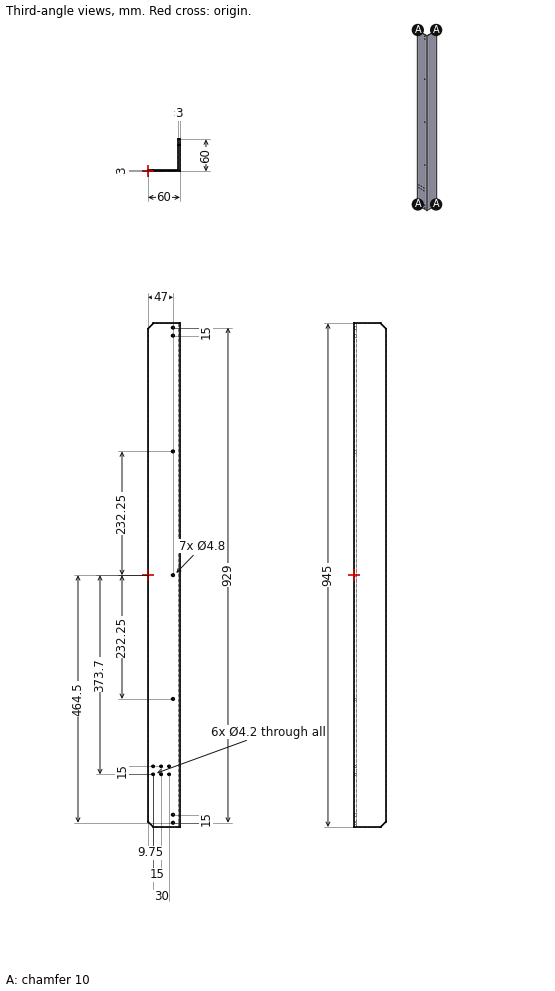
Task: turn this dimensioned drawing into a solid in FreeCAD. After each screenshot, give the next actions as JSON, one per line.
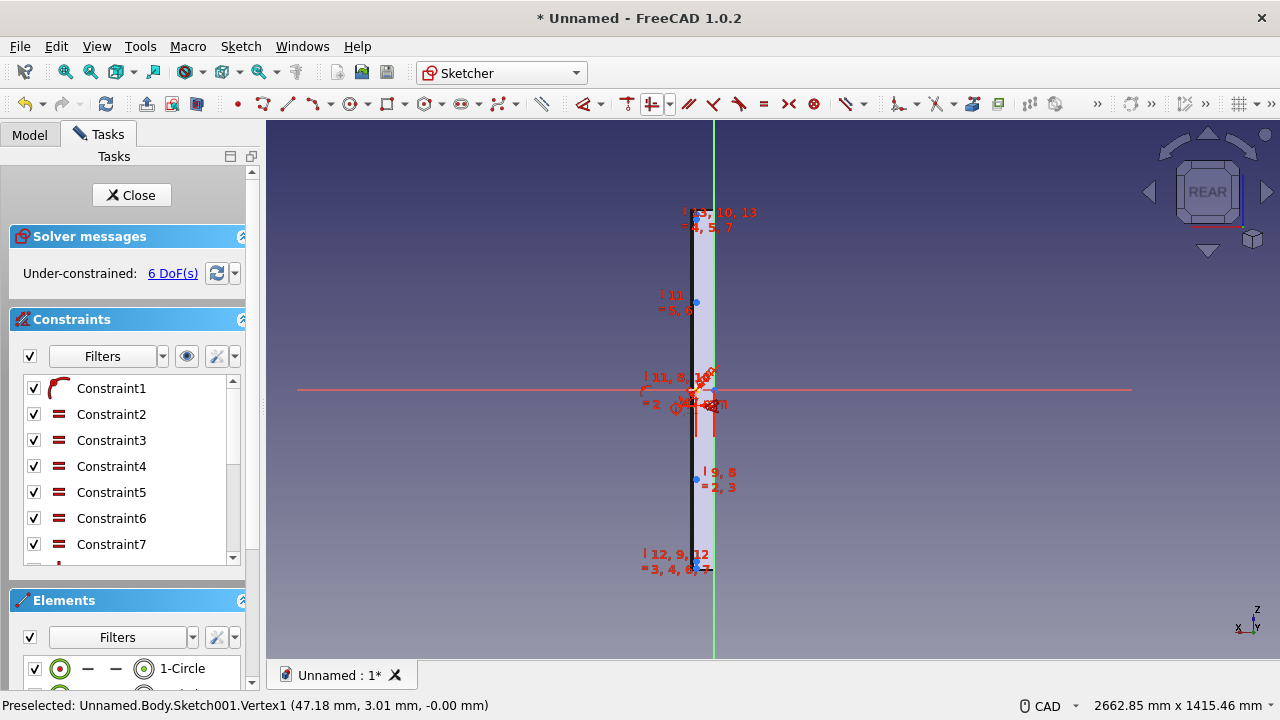
{"action": "scroll", "coordinate": [696, 568], "scroll_direction": "up", "scroll_amount": 10}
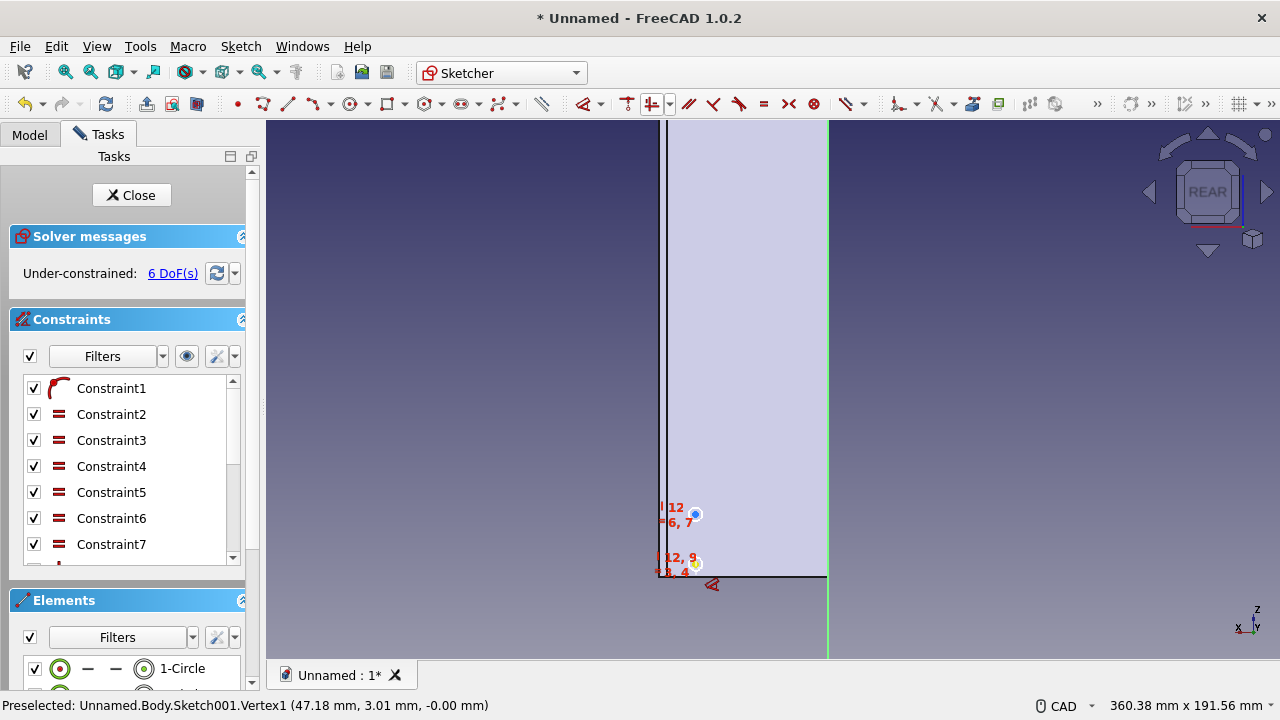
{"action": "left_click", "coordinate": [696, 564]}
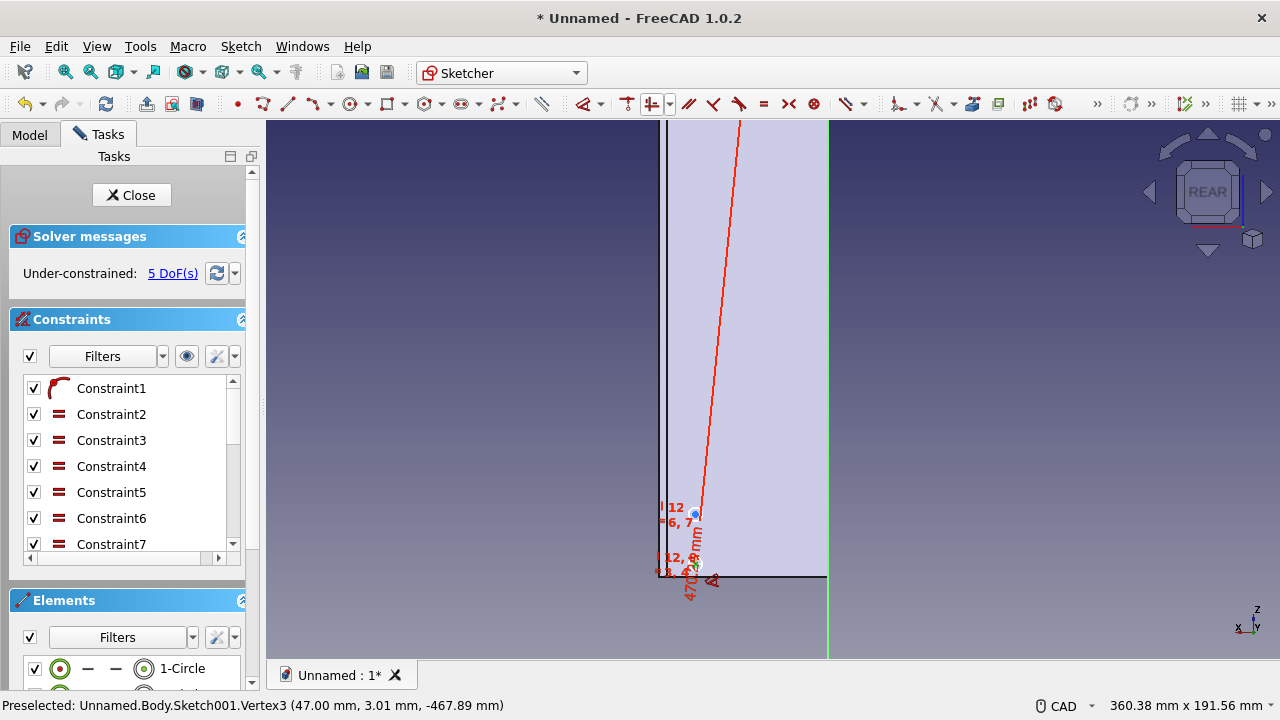
{"action": "left_click", "coordinate": [696, 514]}
{"action": "left_click", "coordinate": [662, 539]}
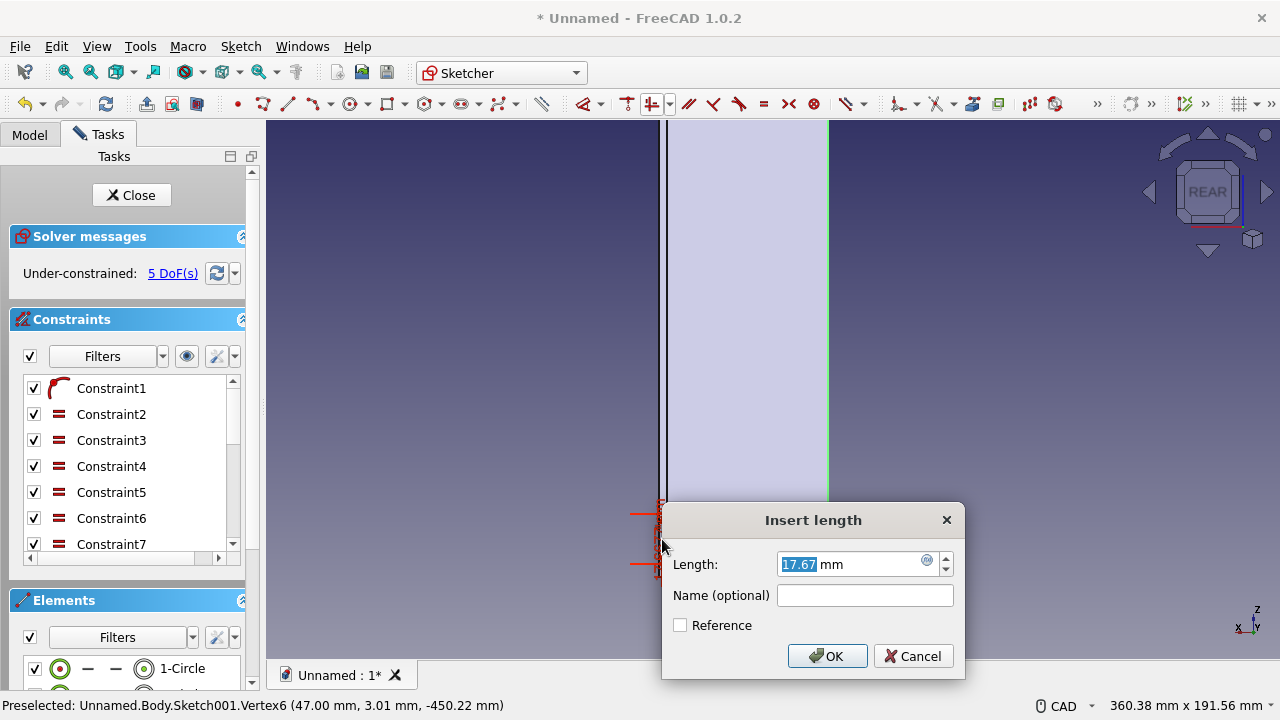
{"action": "type", "text": "15"}
{"action": "key", "text": "Return"}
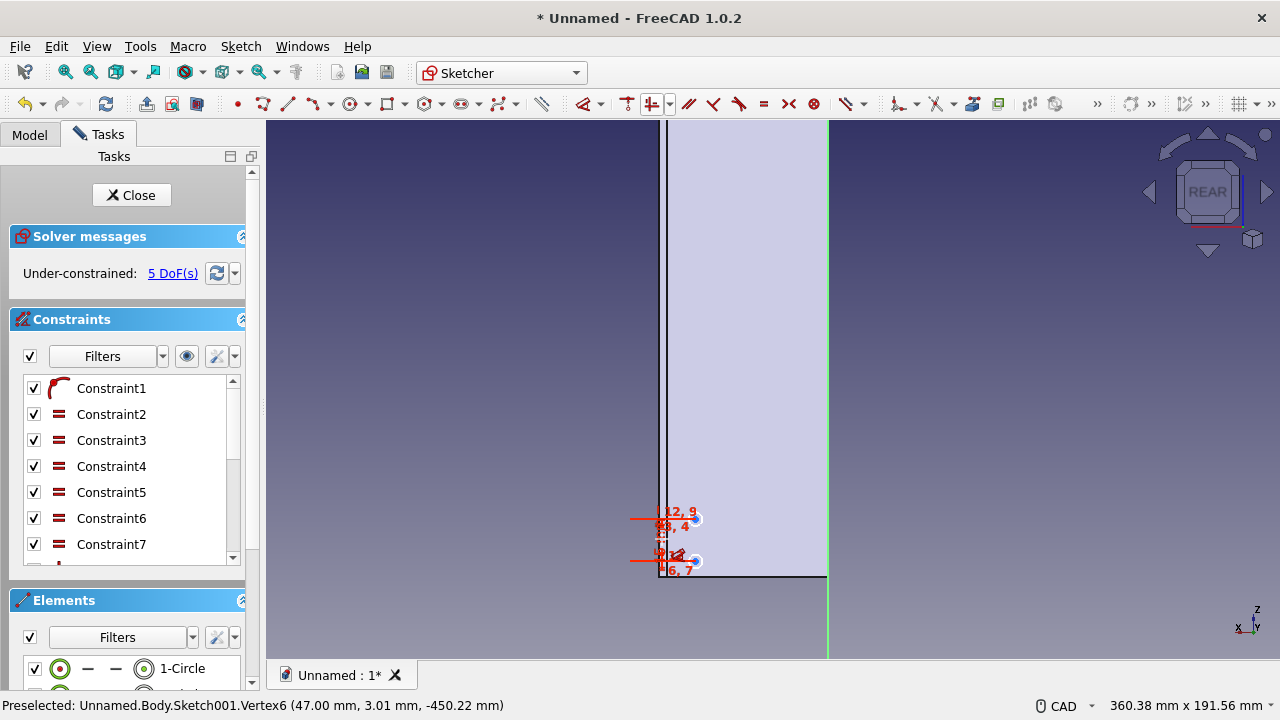
{"action": "scroll", "coordinate": [696, 568], "scroll_direction": "down", "scroll_amount": 10}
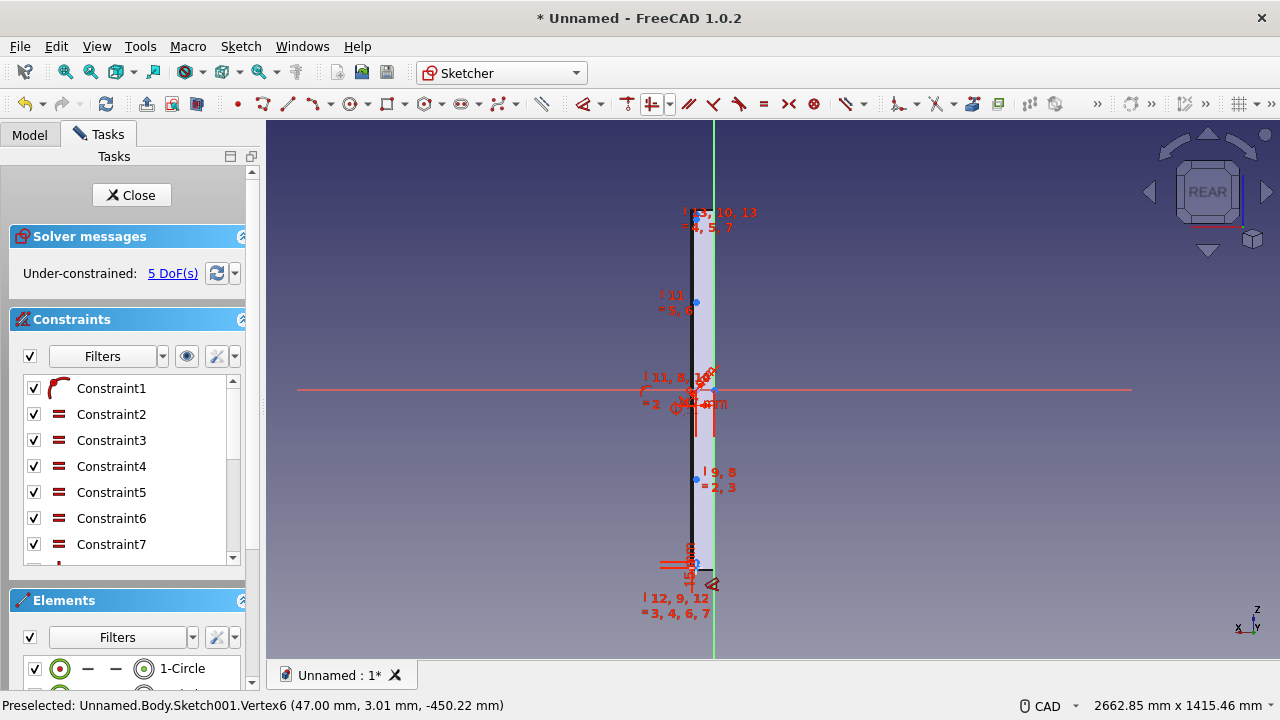
{"action": "scroll", "coordinate": [696, 214], "scroll_direction": "up", "scroll_amount": 10}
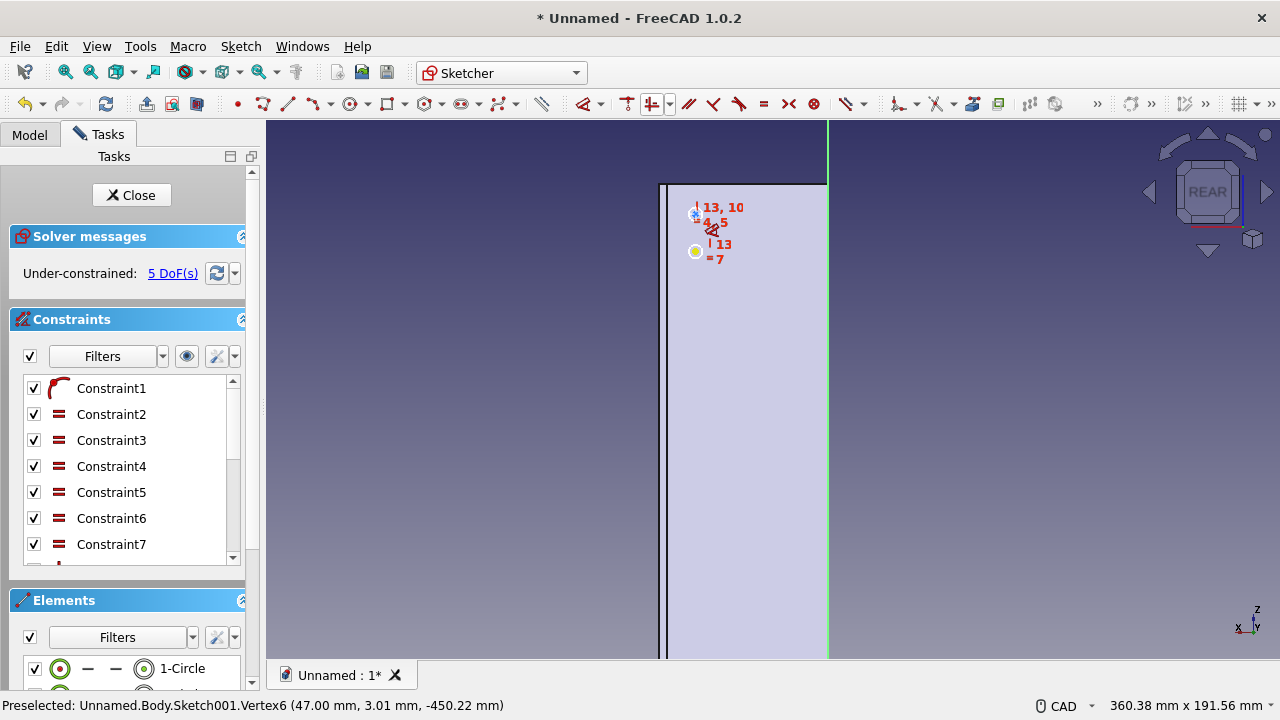
{"action": "left_click", "coordinate": [696, 214]}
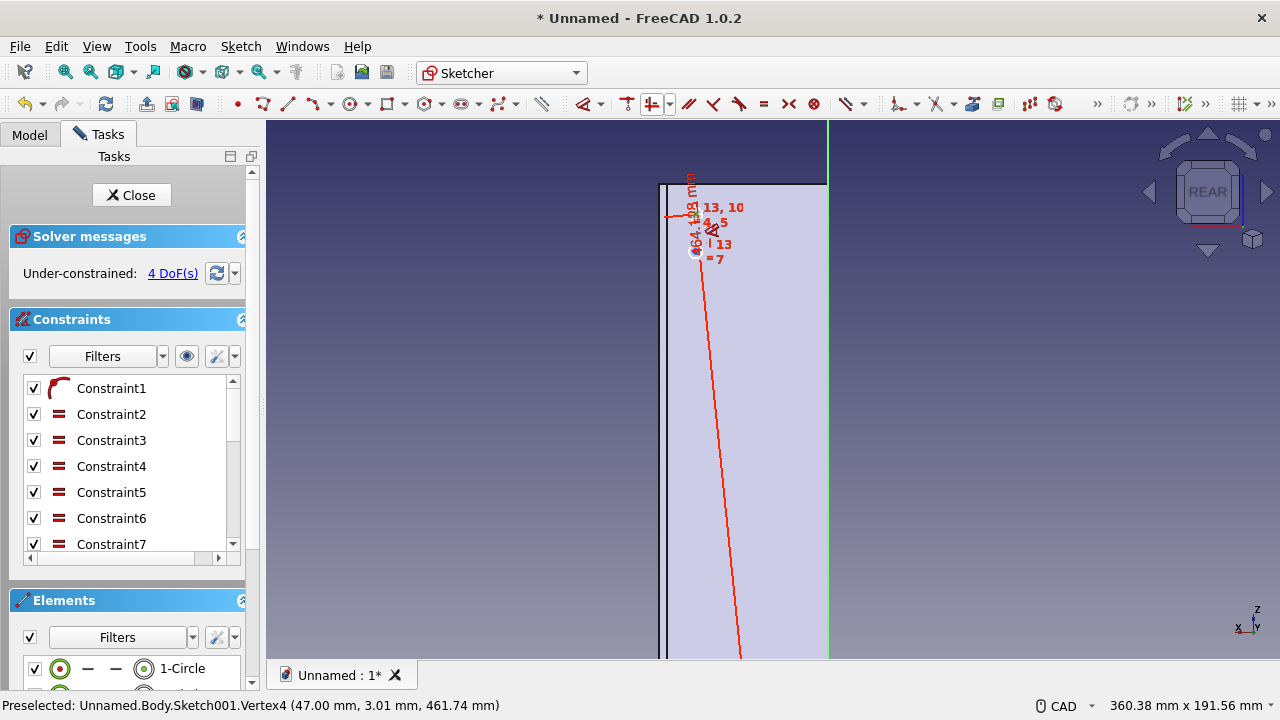
{"action": "left_click", "coordinate": [696, 252]}
{"action": "left_click", "coordinate": [662, 233]}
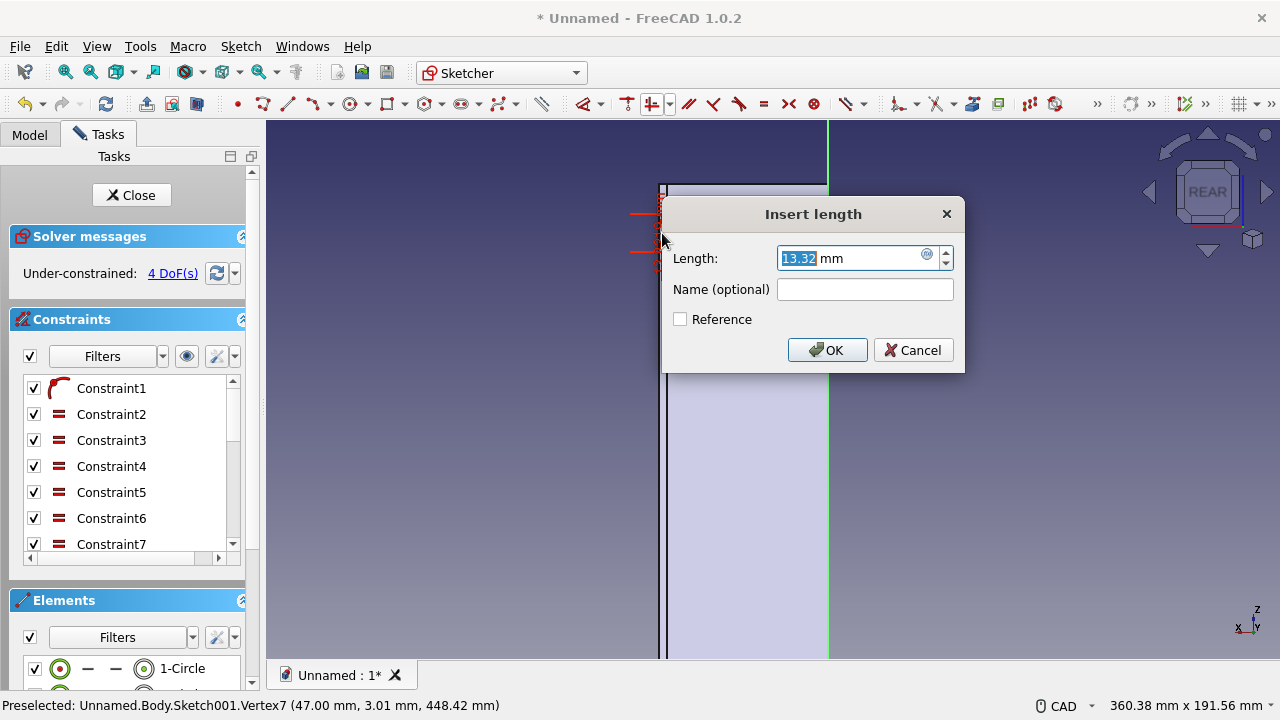
{"action": "type", "text": "15"}
{"action": "key", "text": "Return"}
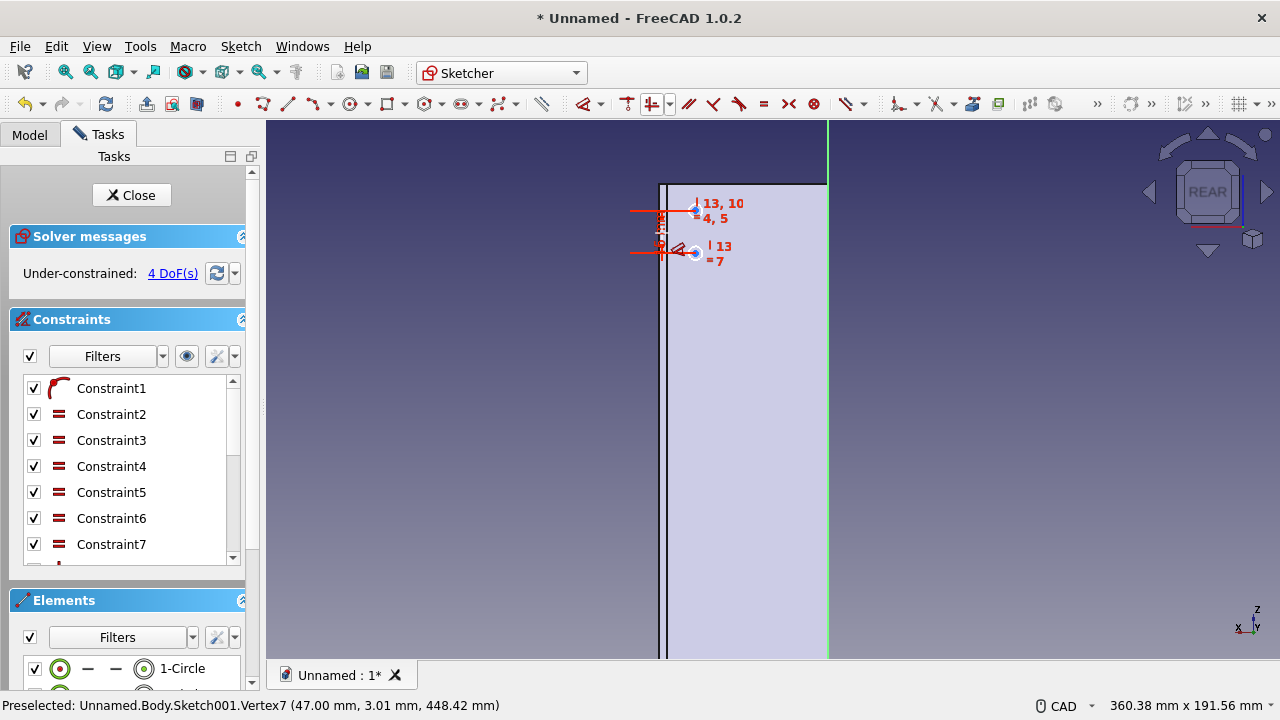
{"action": "scroll", "coordinate": [696, 214], "scroll_direction": "down", "scroll_amount": 10}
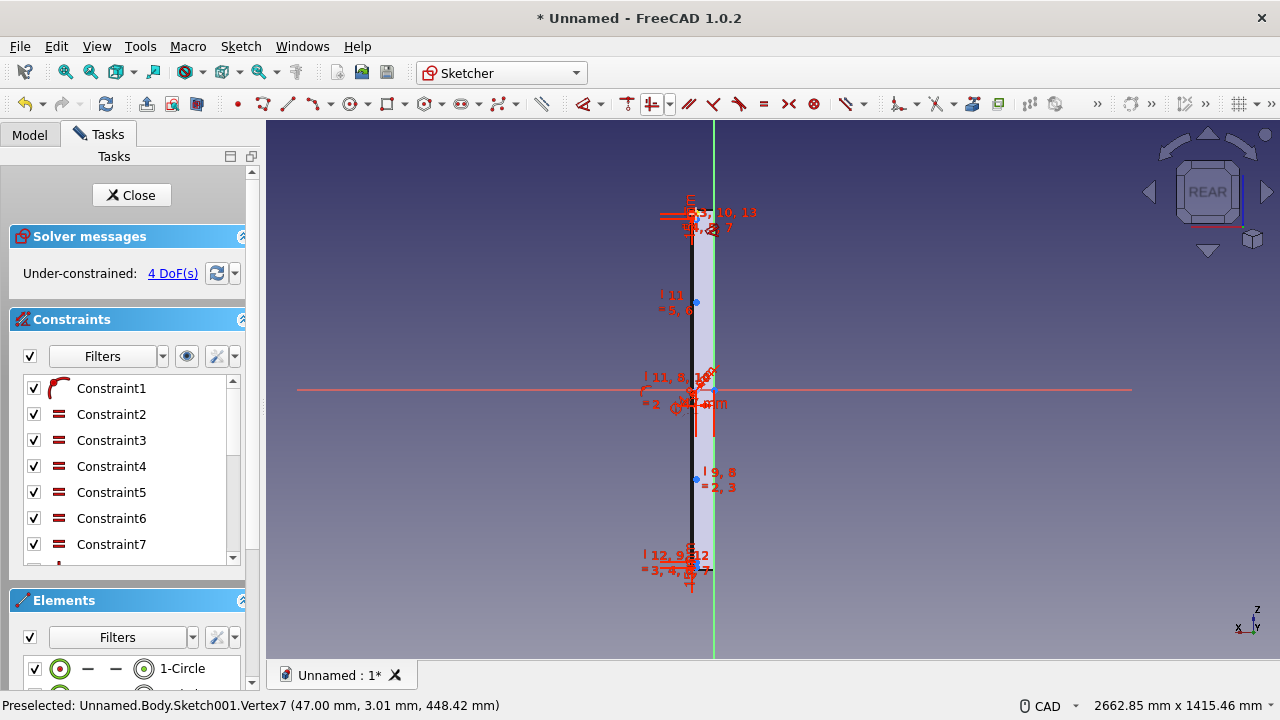
{"action": "scroll", "coordinate": [696, 568], "scroll_direction": "up", "scroll_amount": 4}